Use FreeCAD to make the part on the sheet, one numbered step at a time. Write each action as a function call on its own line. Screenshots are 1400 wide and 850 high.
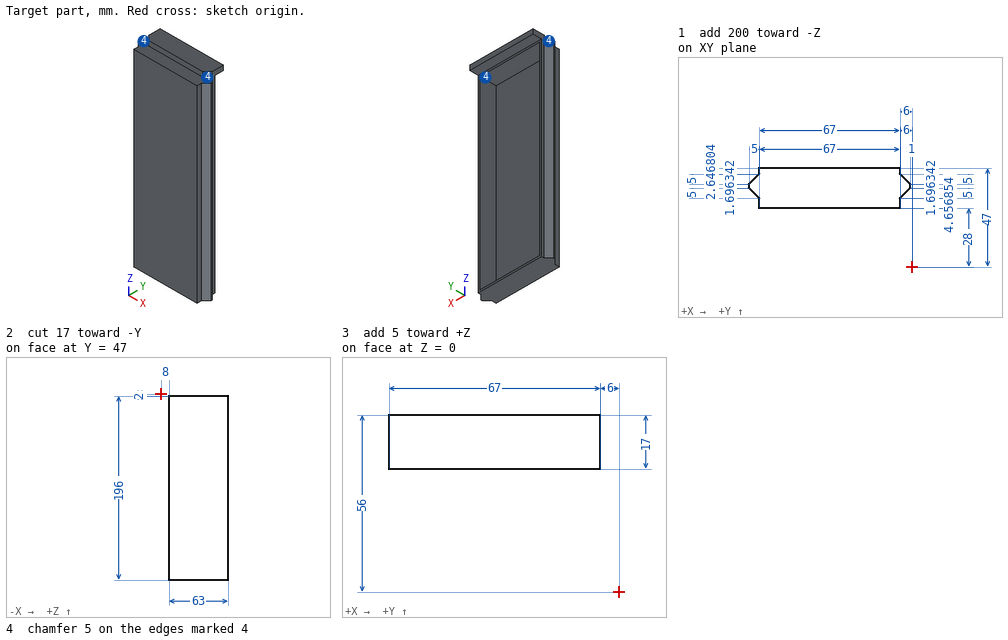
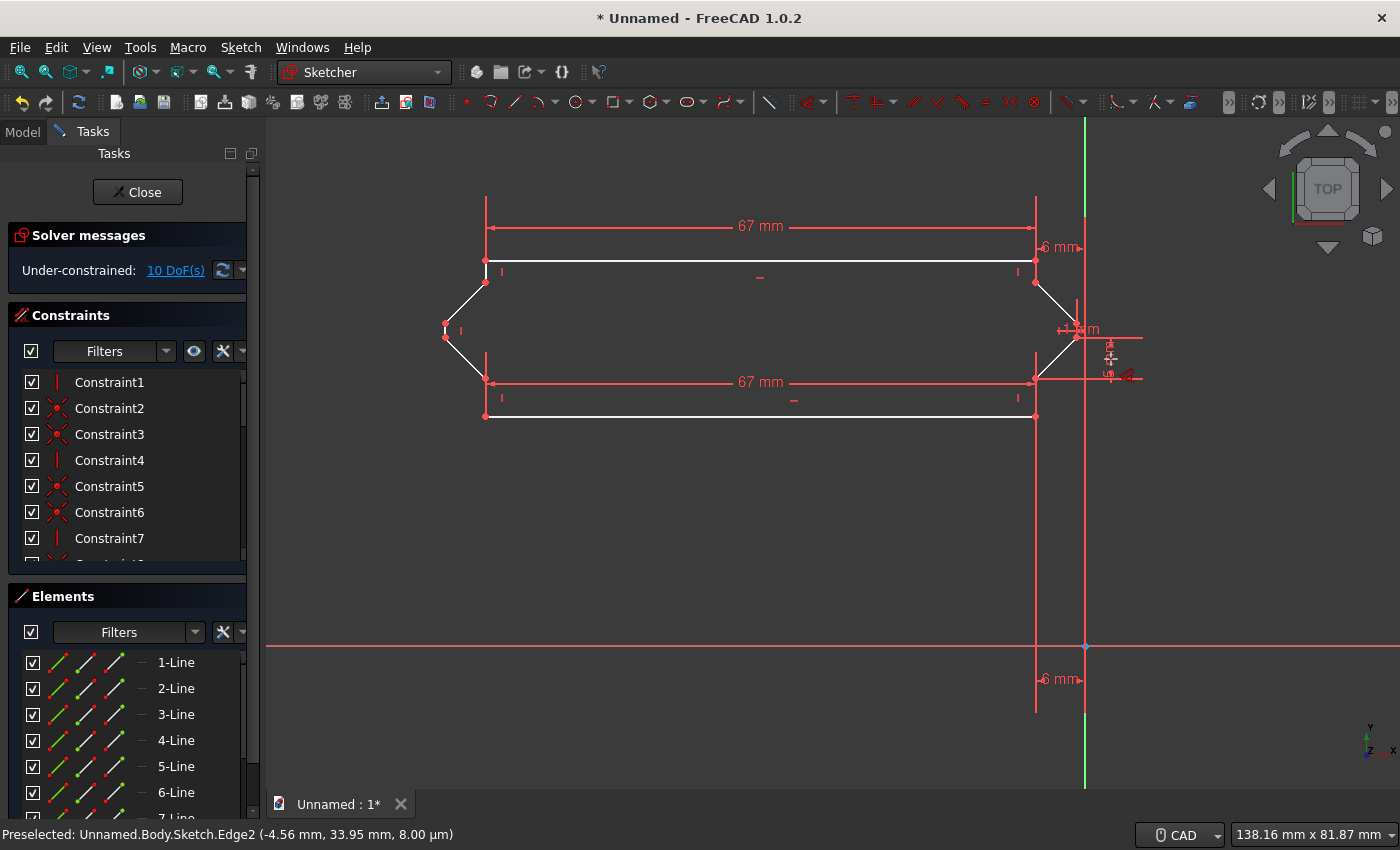
click(1064, 311)
click(1111, 303)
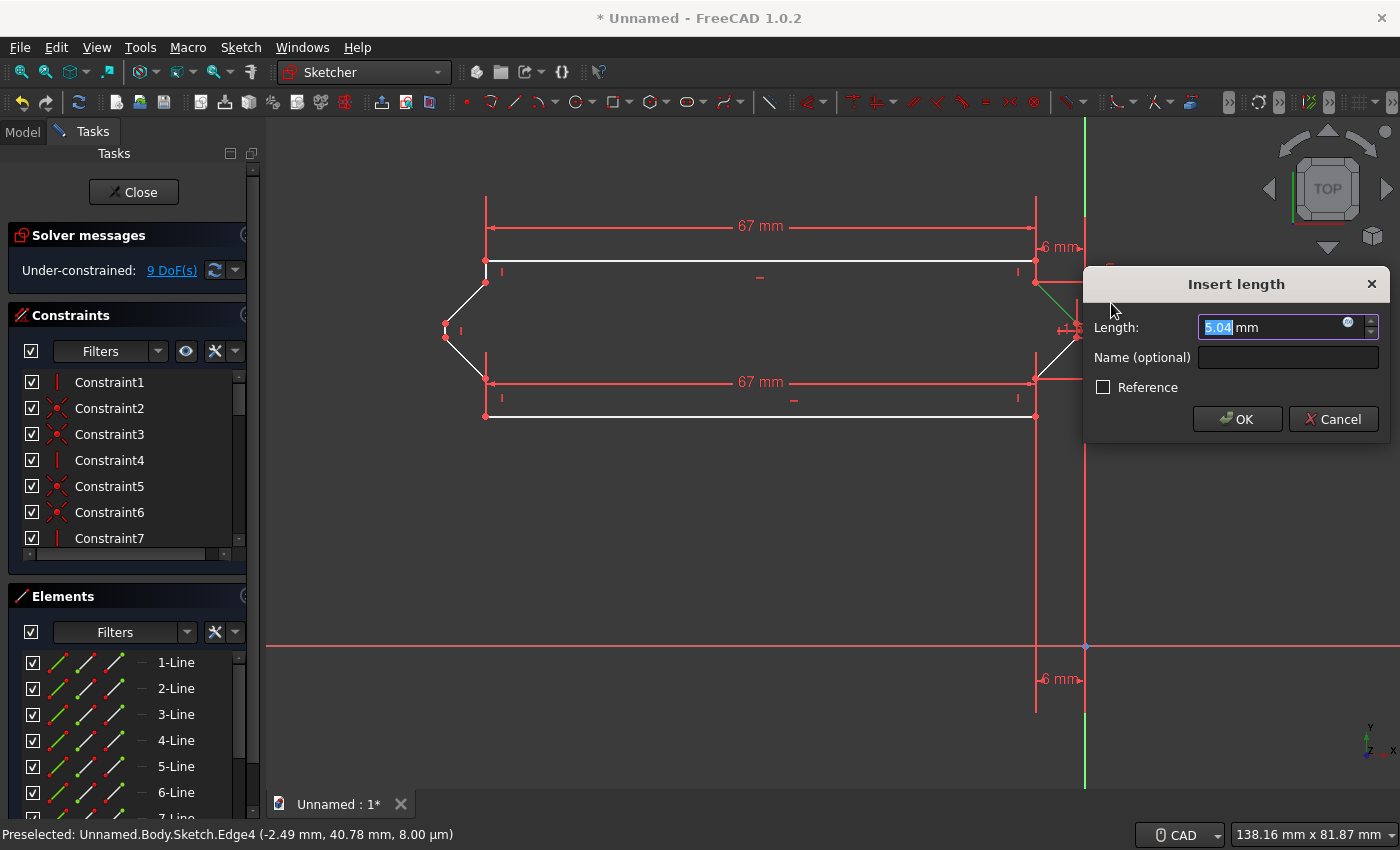
text(5)
key(Return)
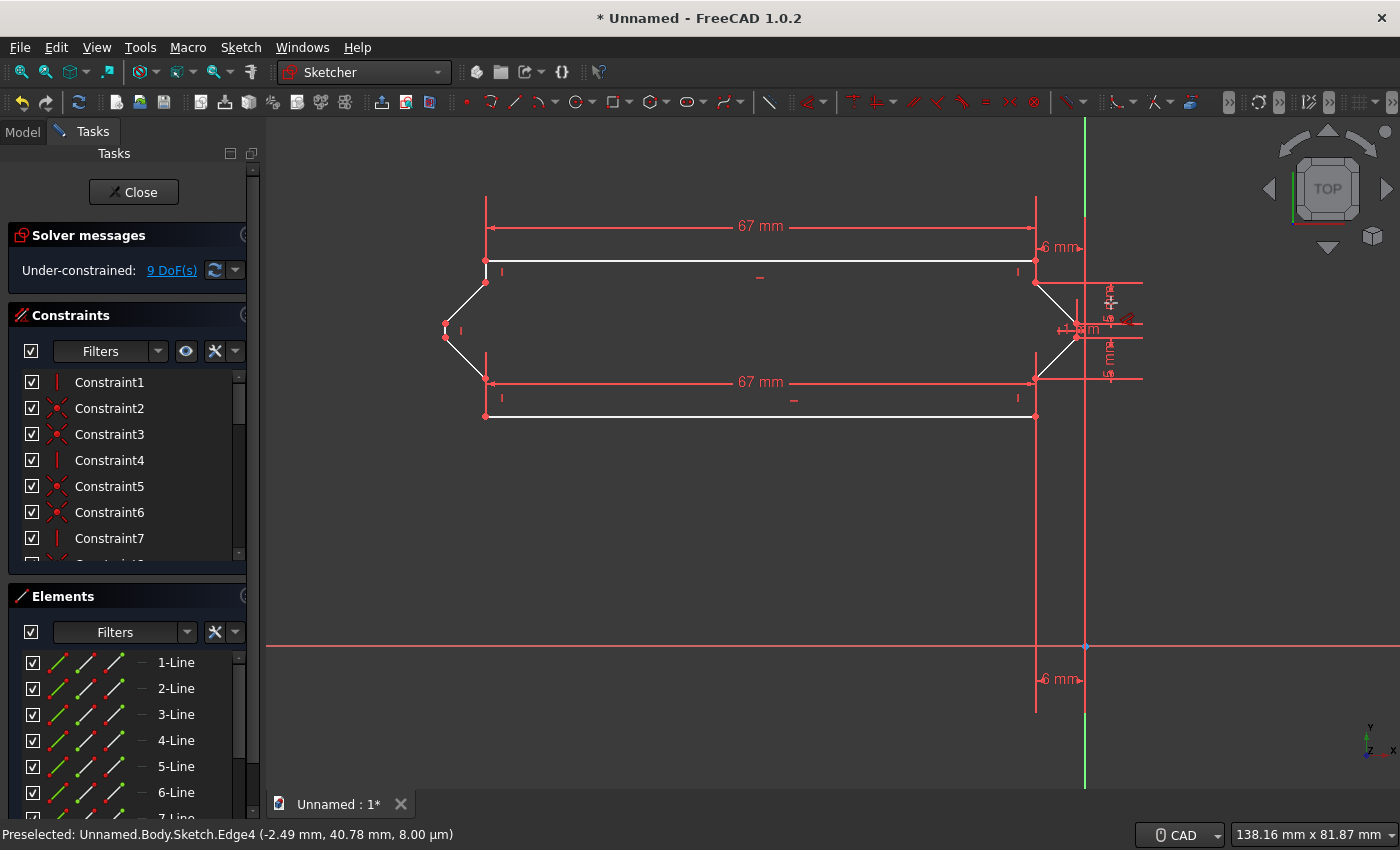
click(474, 295)
click(465, 249)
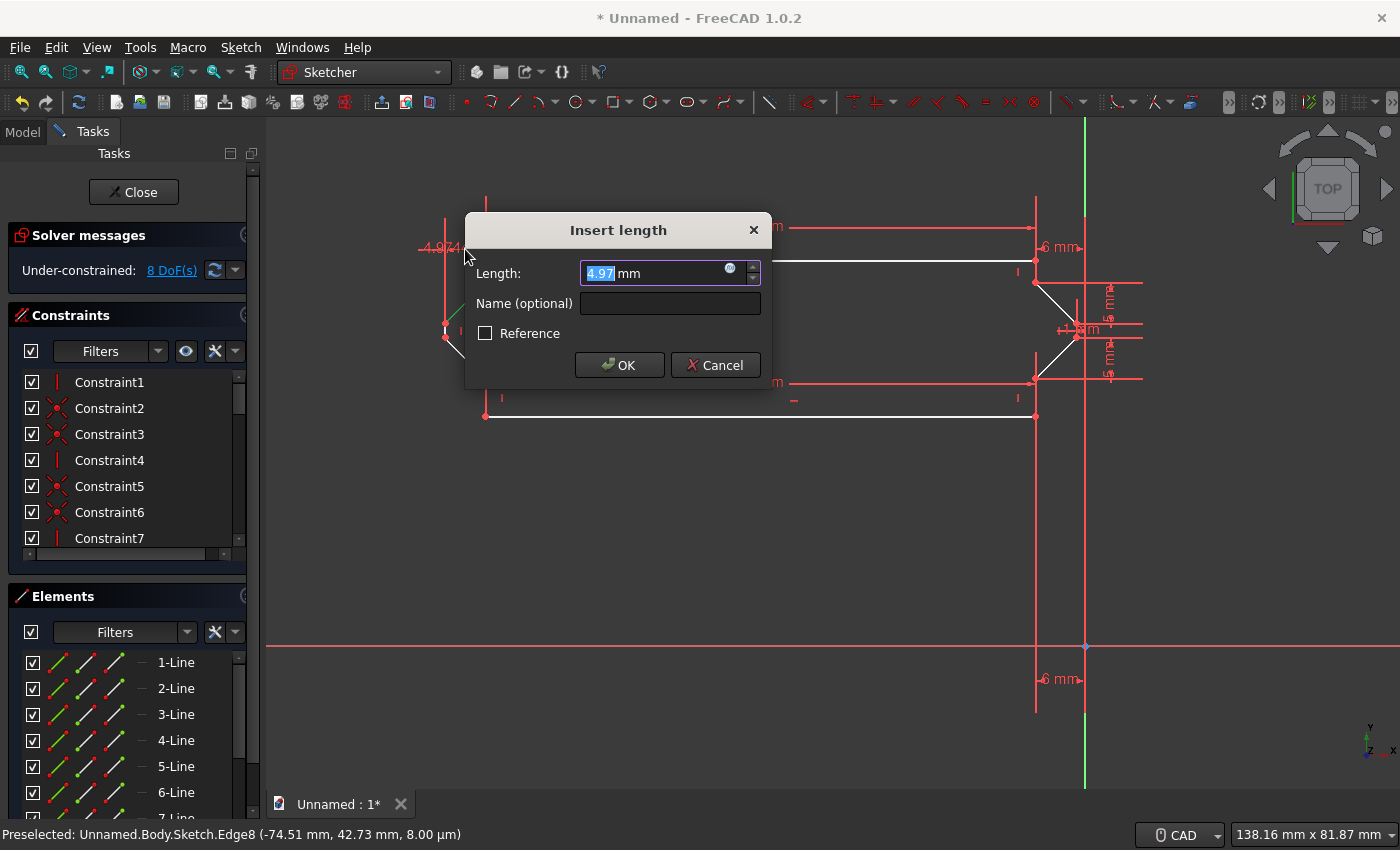
text(5)
key(Return)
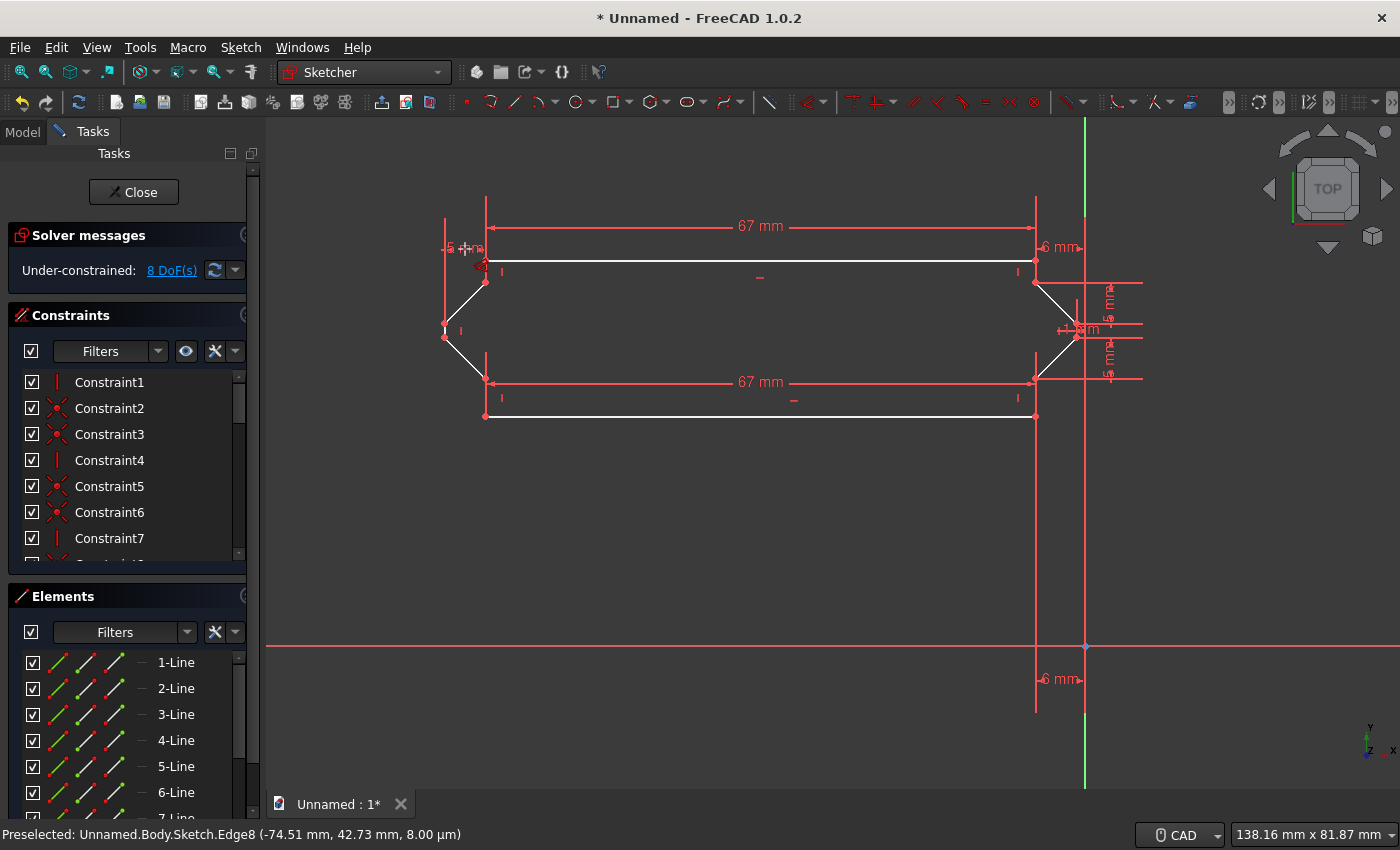
click(474, 295)
click(411, 303)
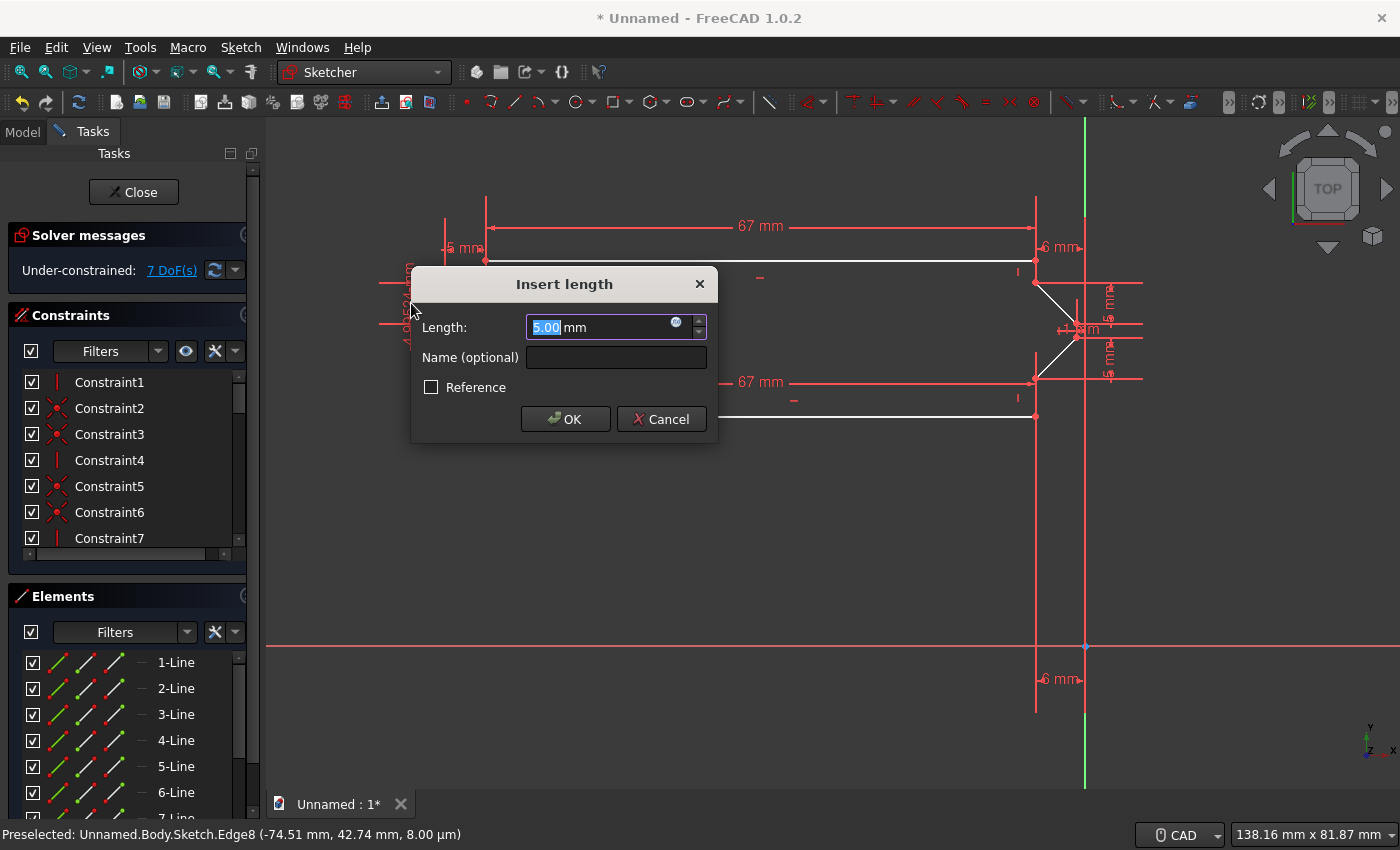
text(5)
key(Return)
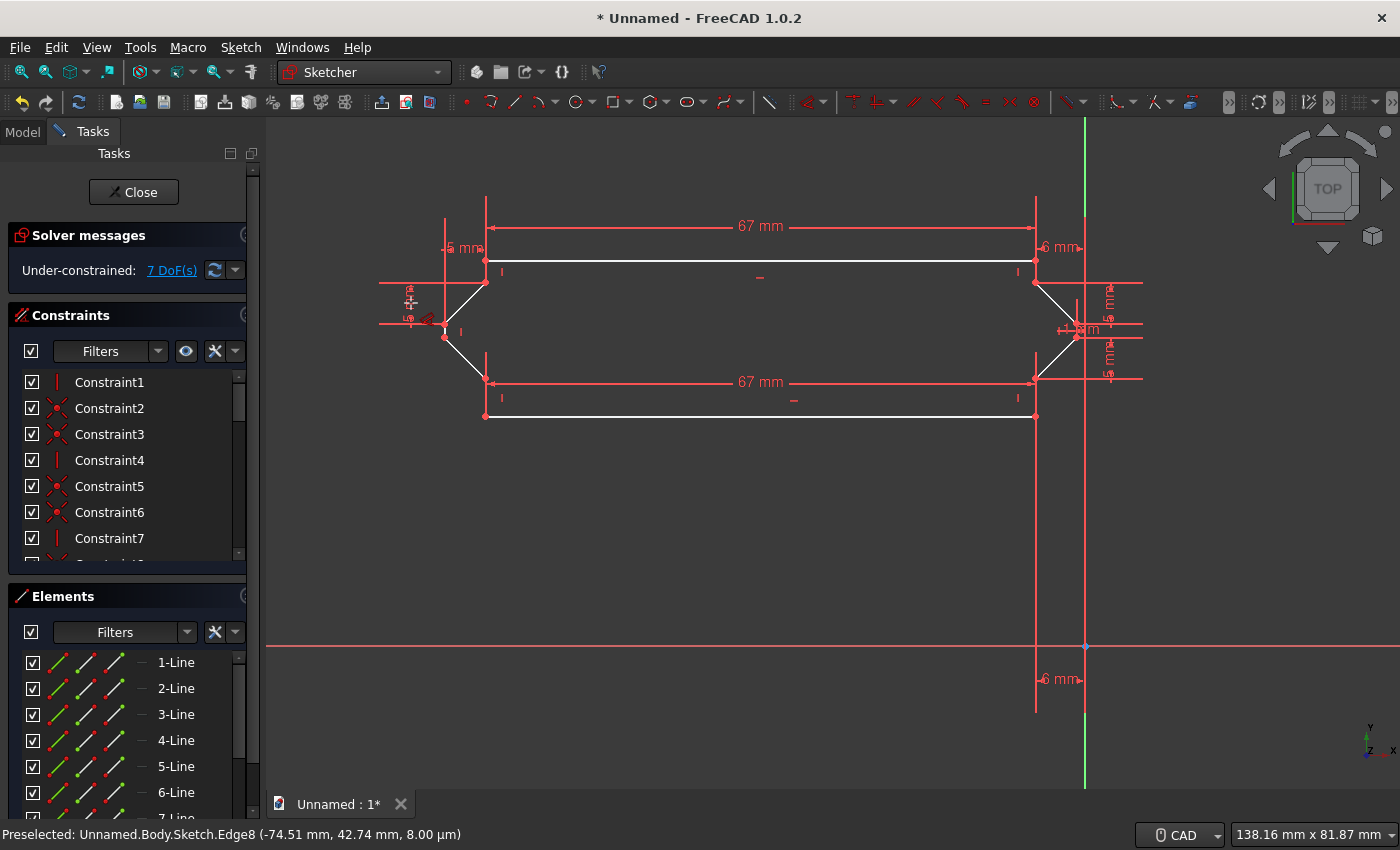
click(457, 350)
click(411, 358)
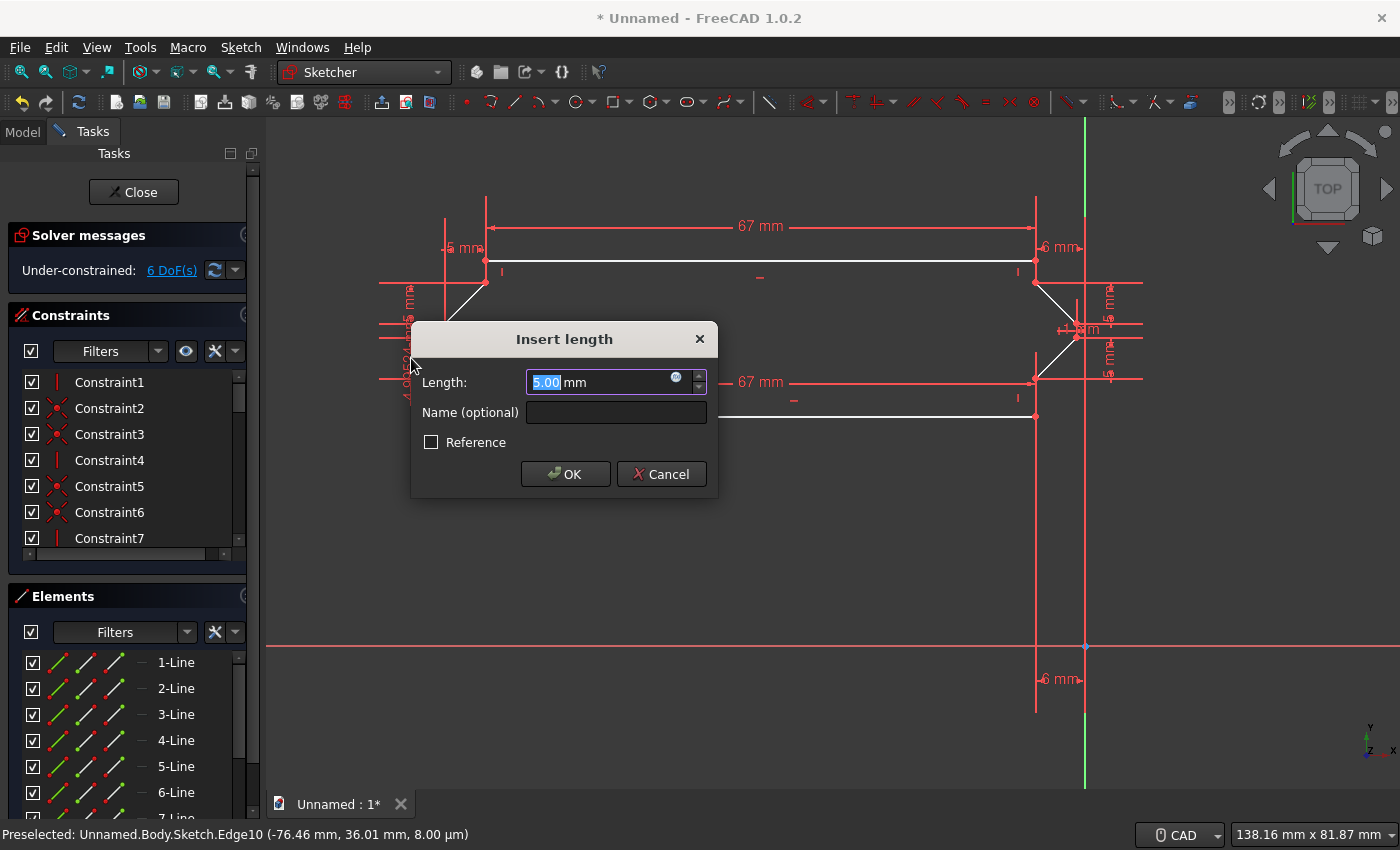
text(5)
key(Return)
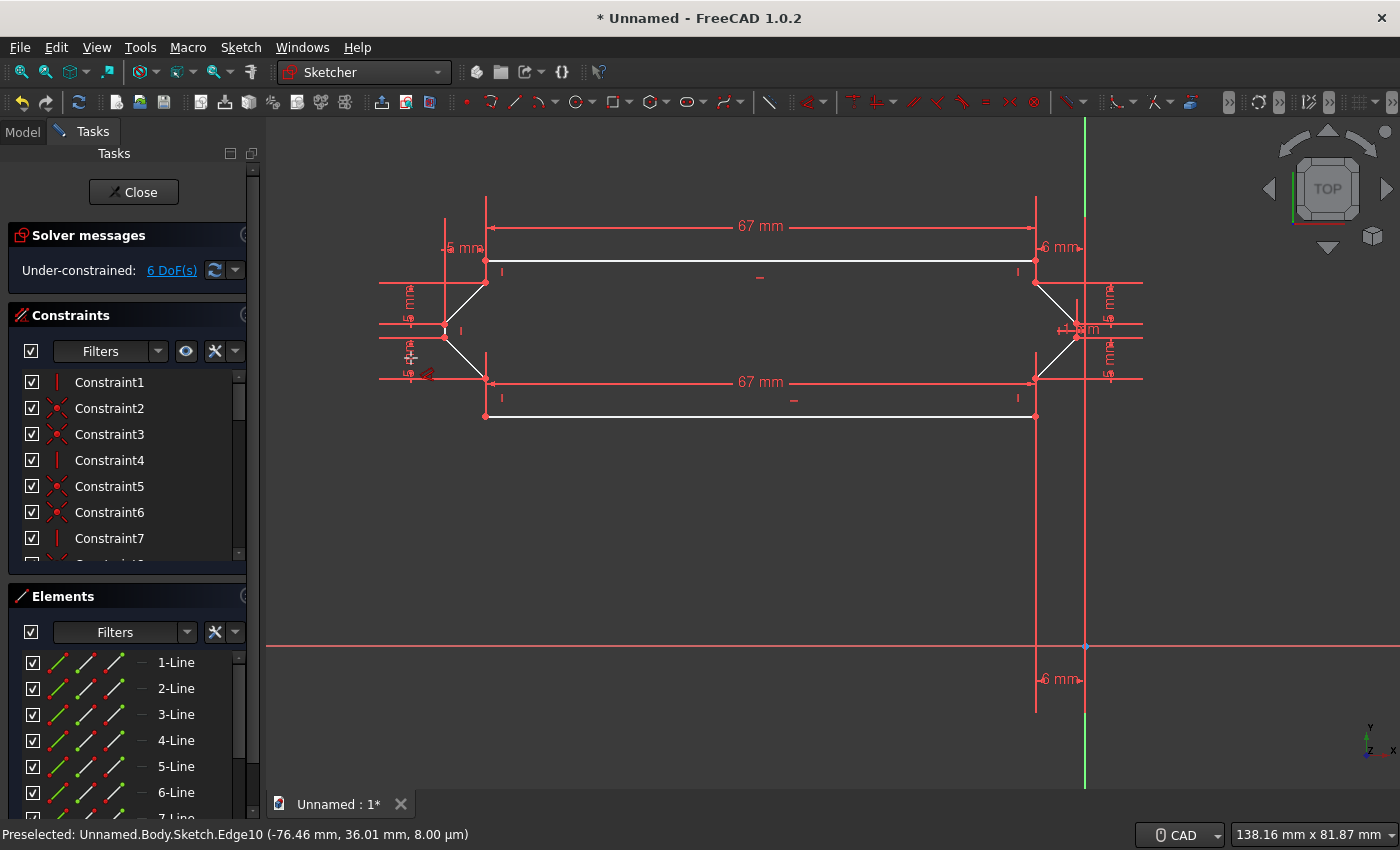
click(1036, 417)
click(1119, 532)